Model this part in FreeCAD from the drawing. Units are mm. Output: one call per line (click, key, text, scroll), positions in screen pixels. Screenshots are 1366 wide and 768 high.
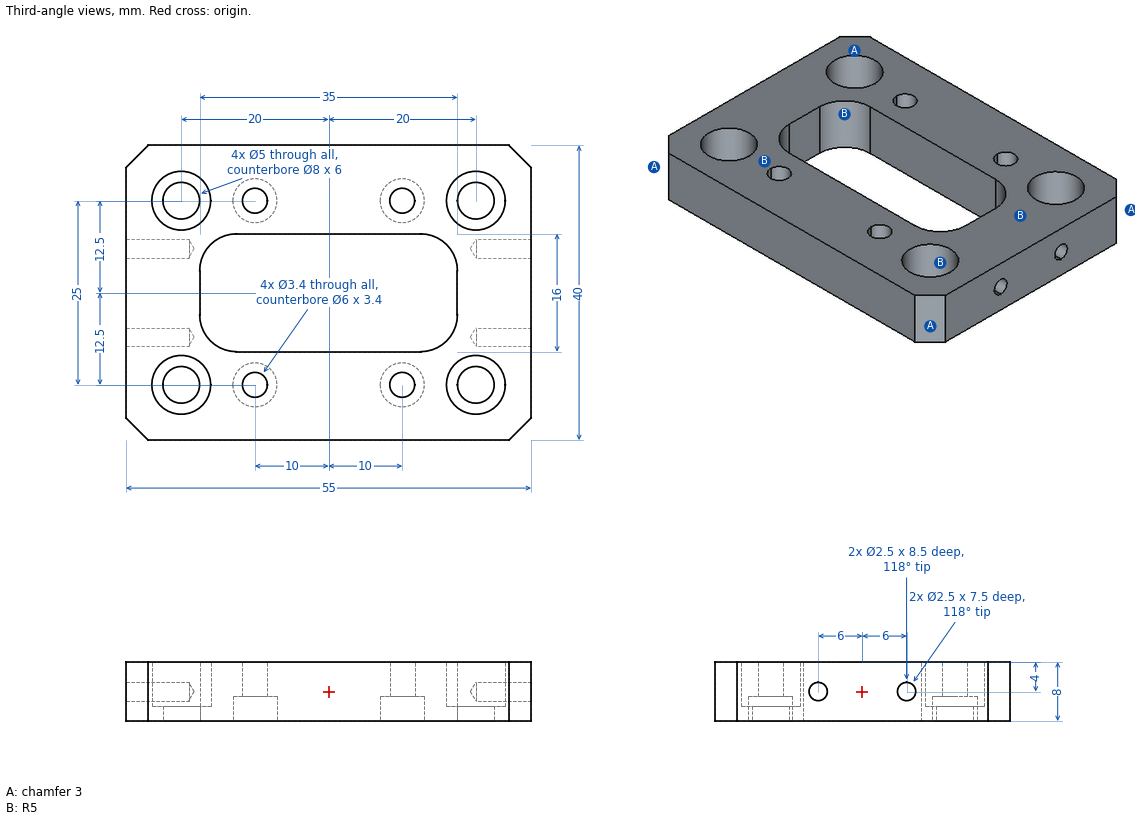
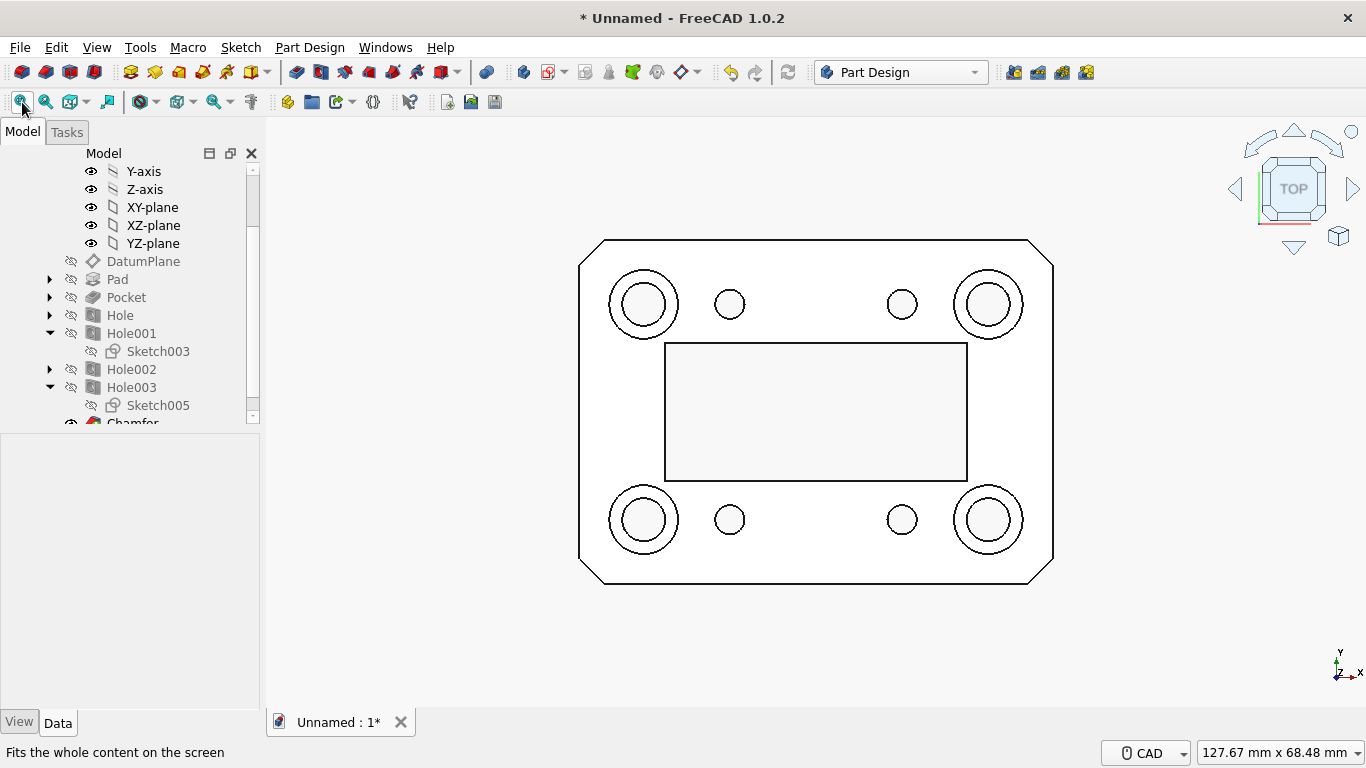
key(1)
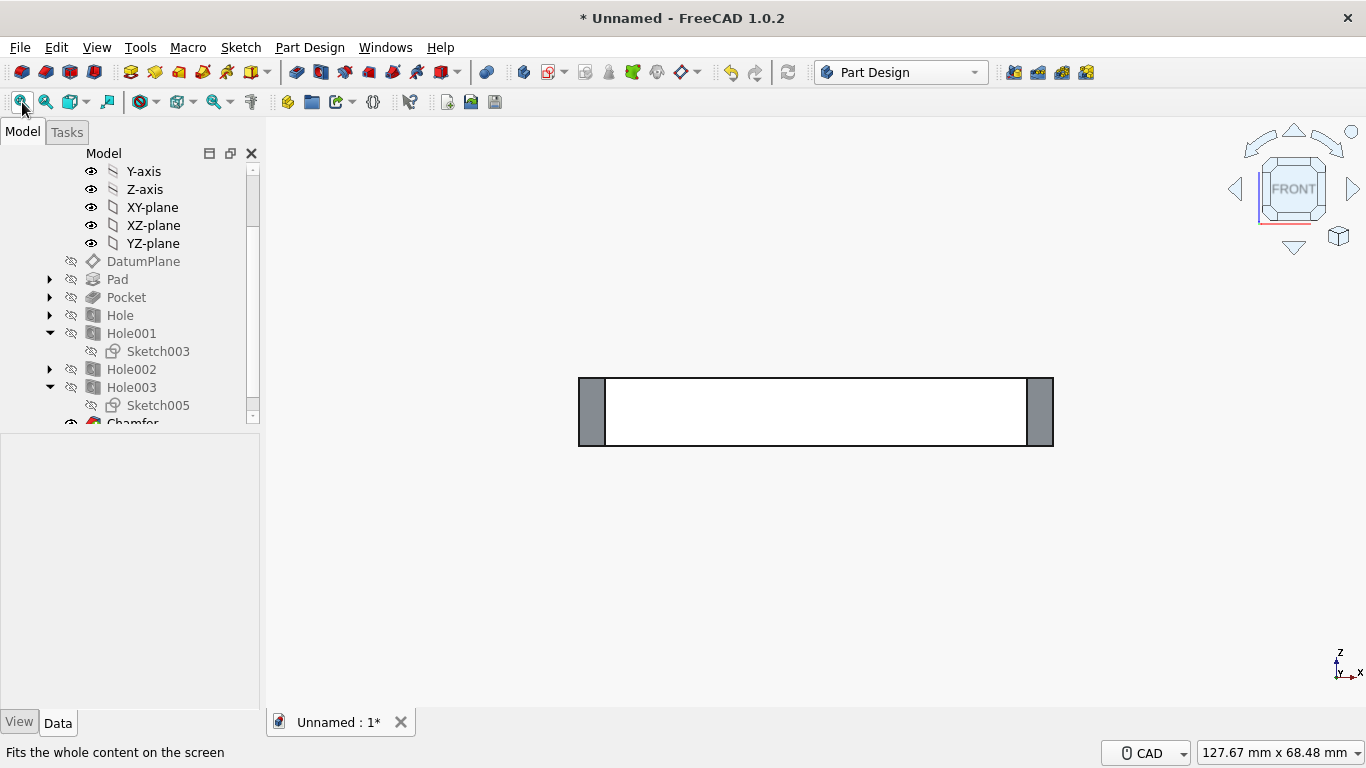
click(22, 102)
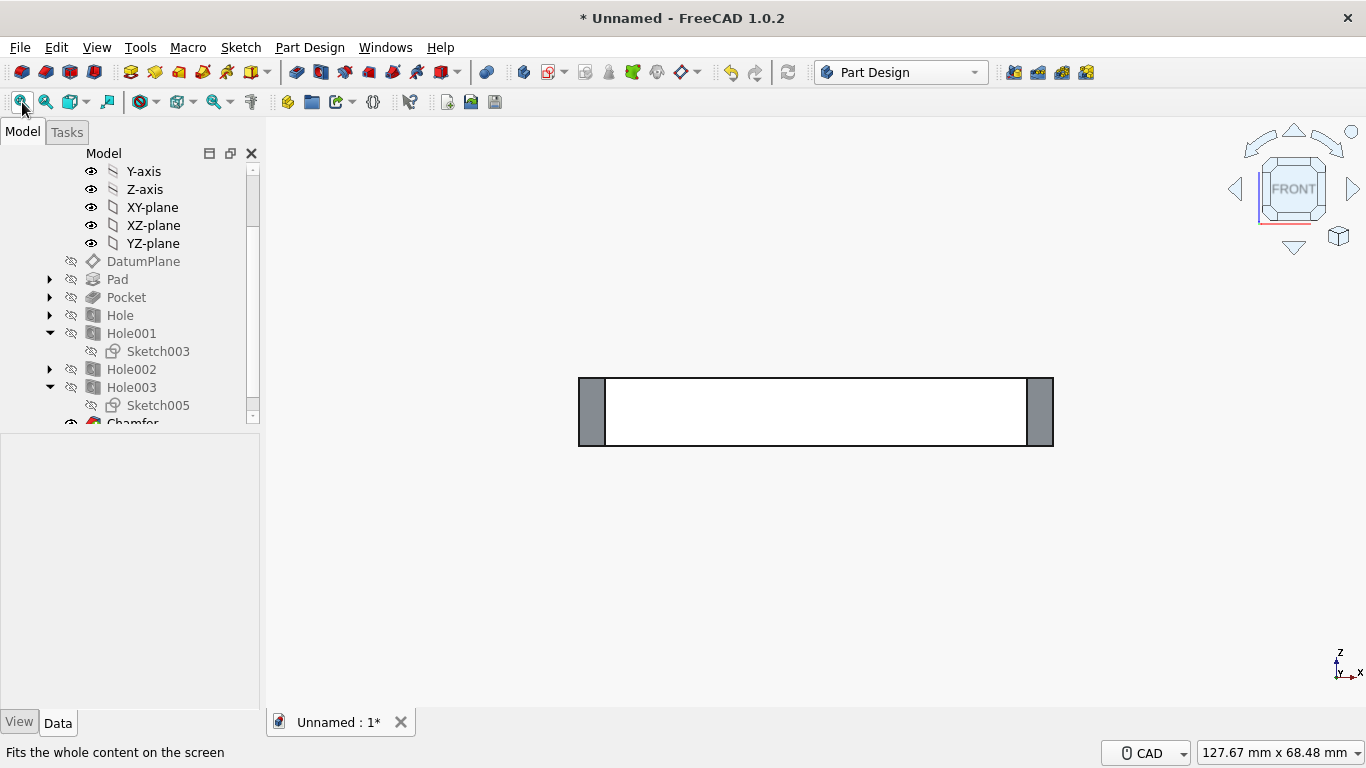
key(3)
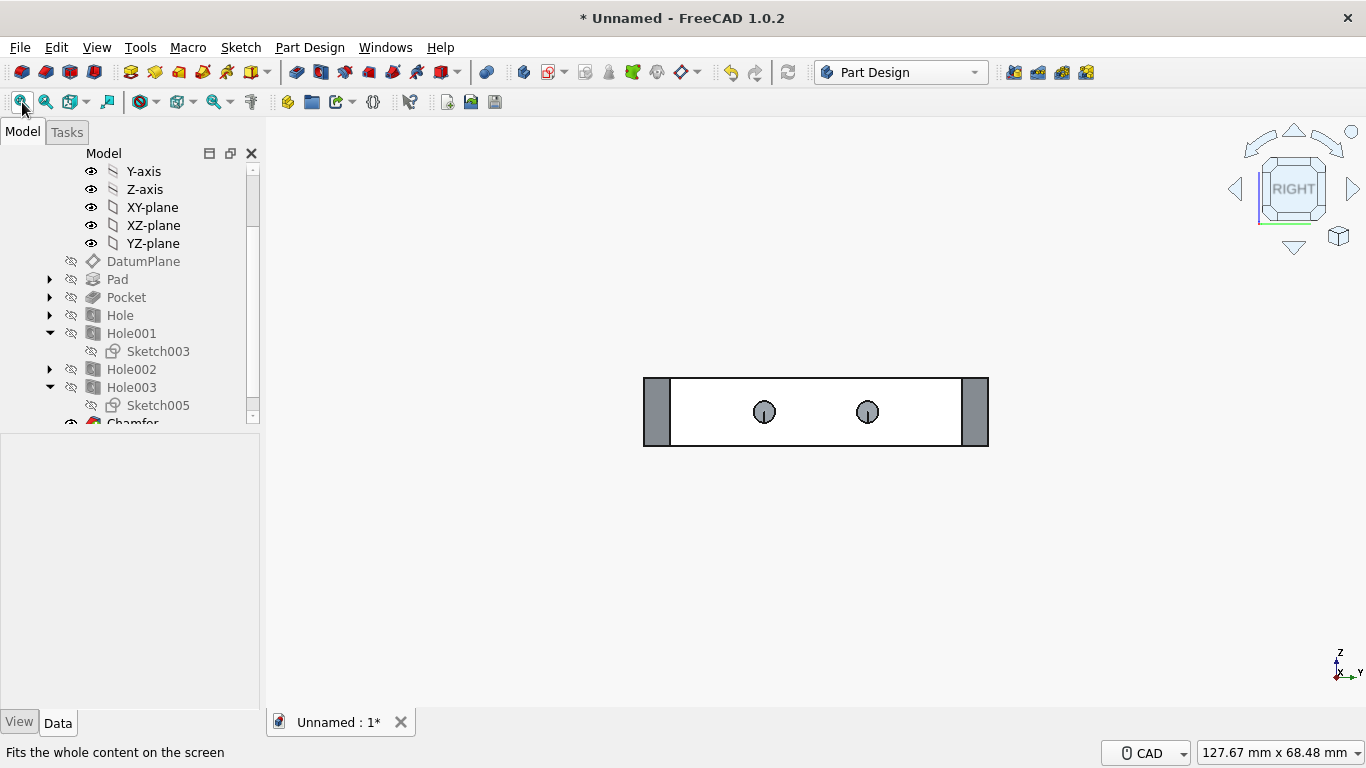
click(22, 102)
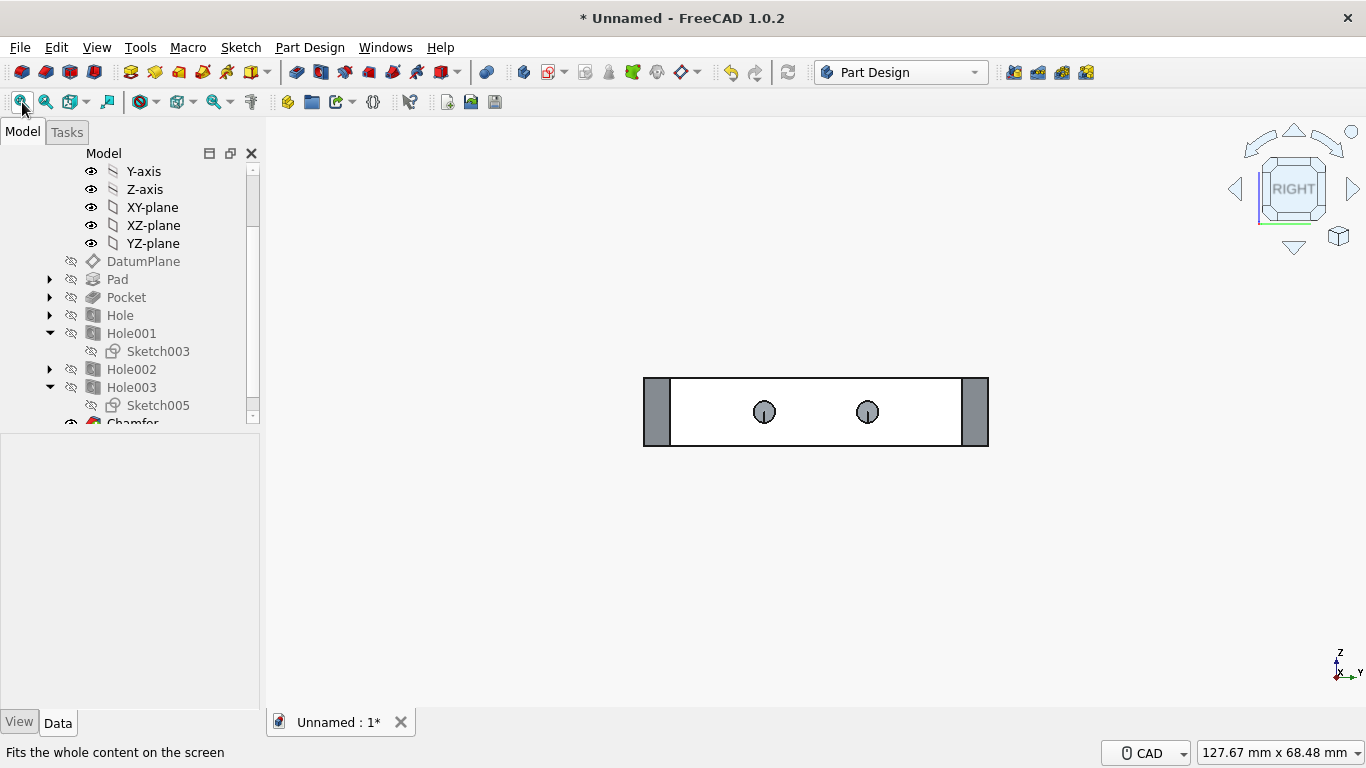
key(5)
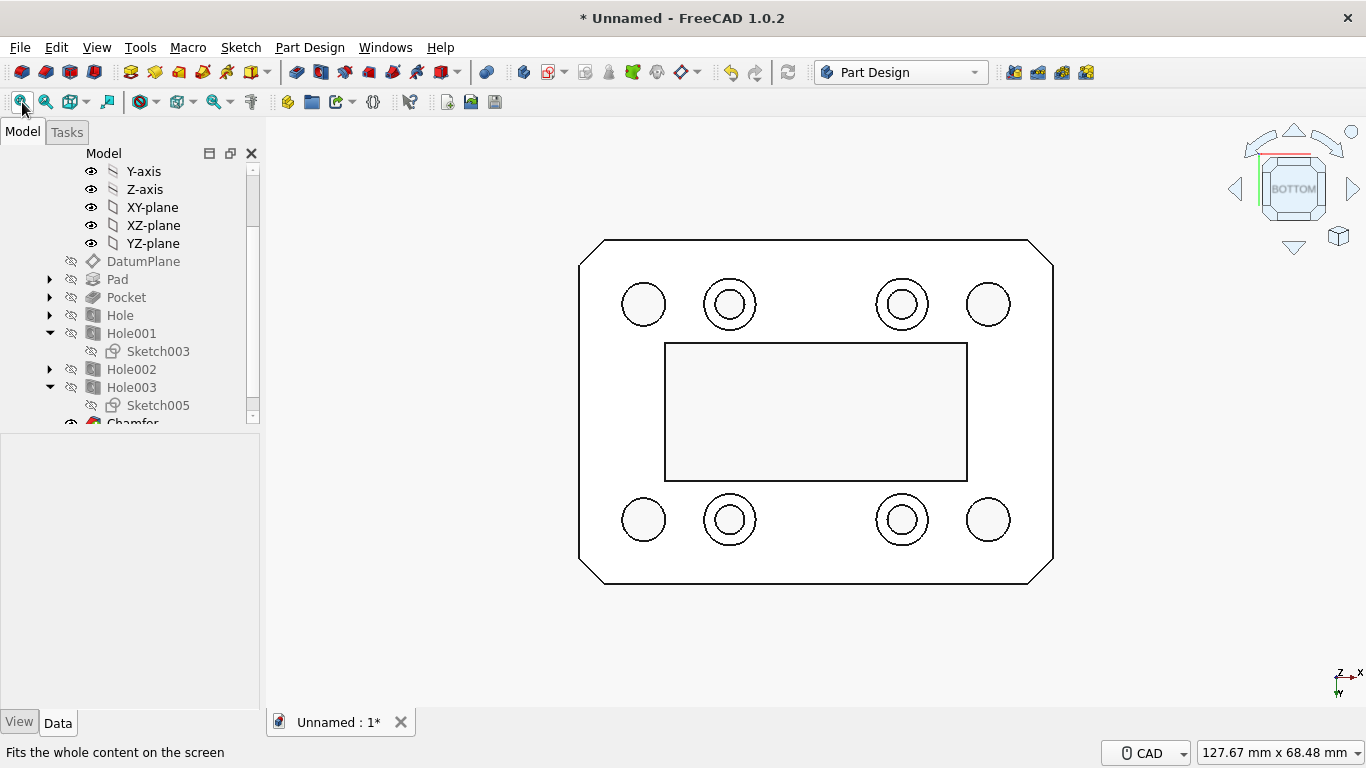
key(4)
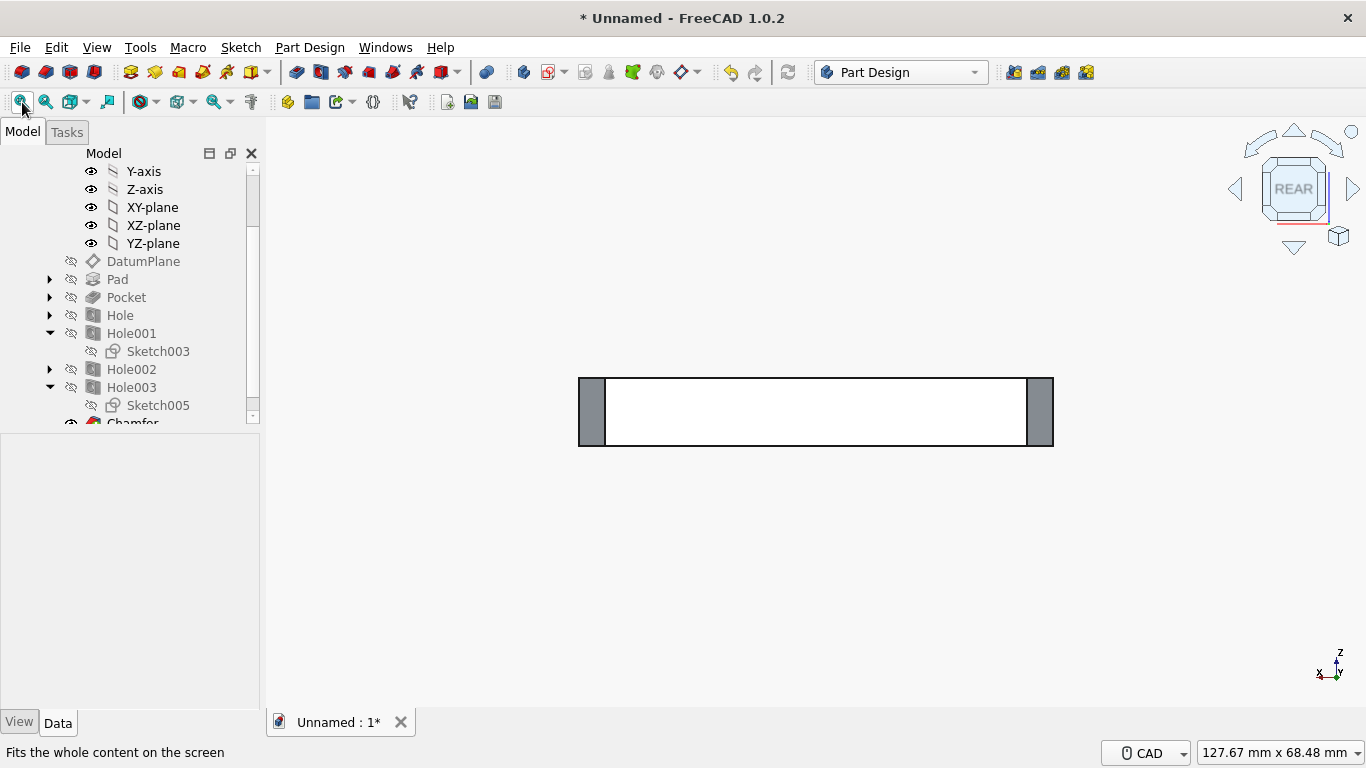
click(22, 102)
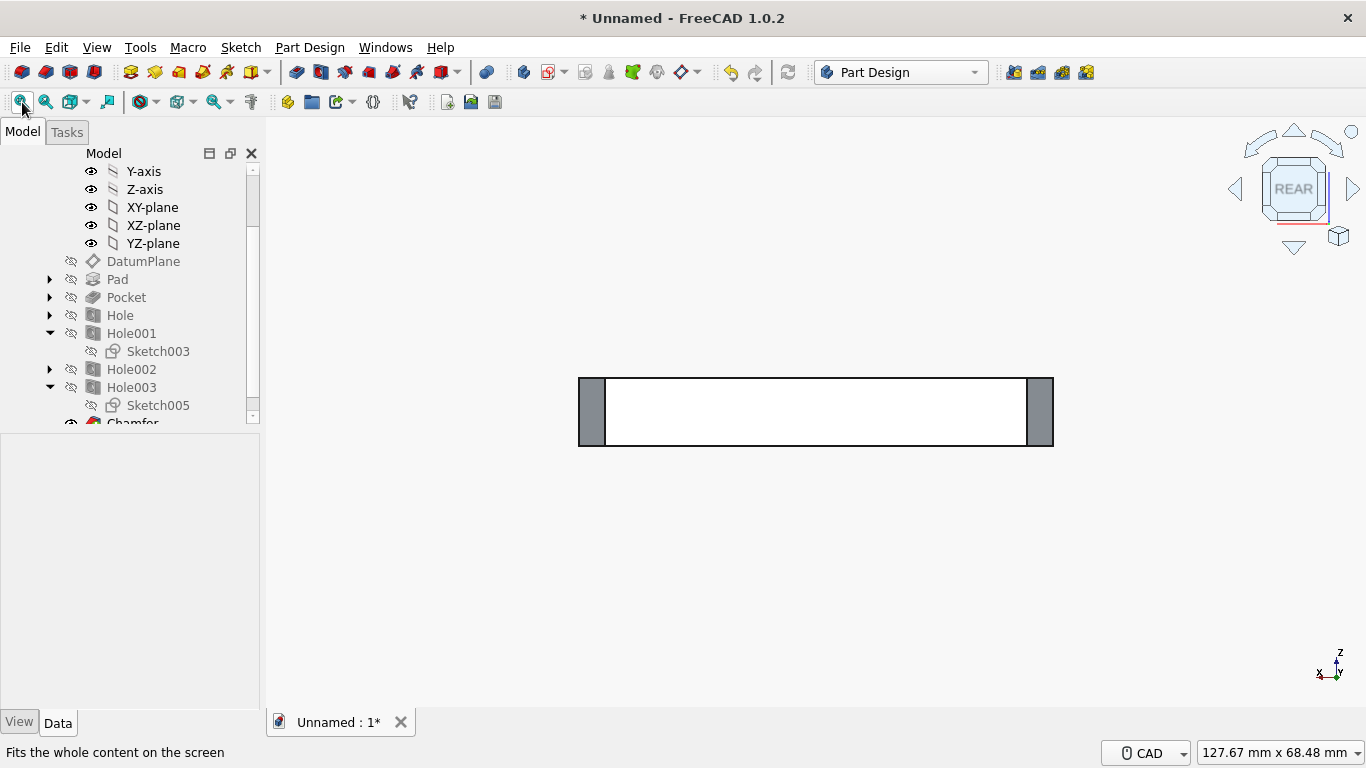
key(6)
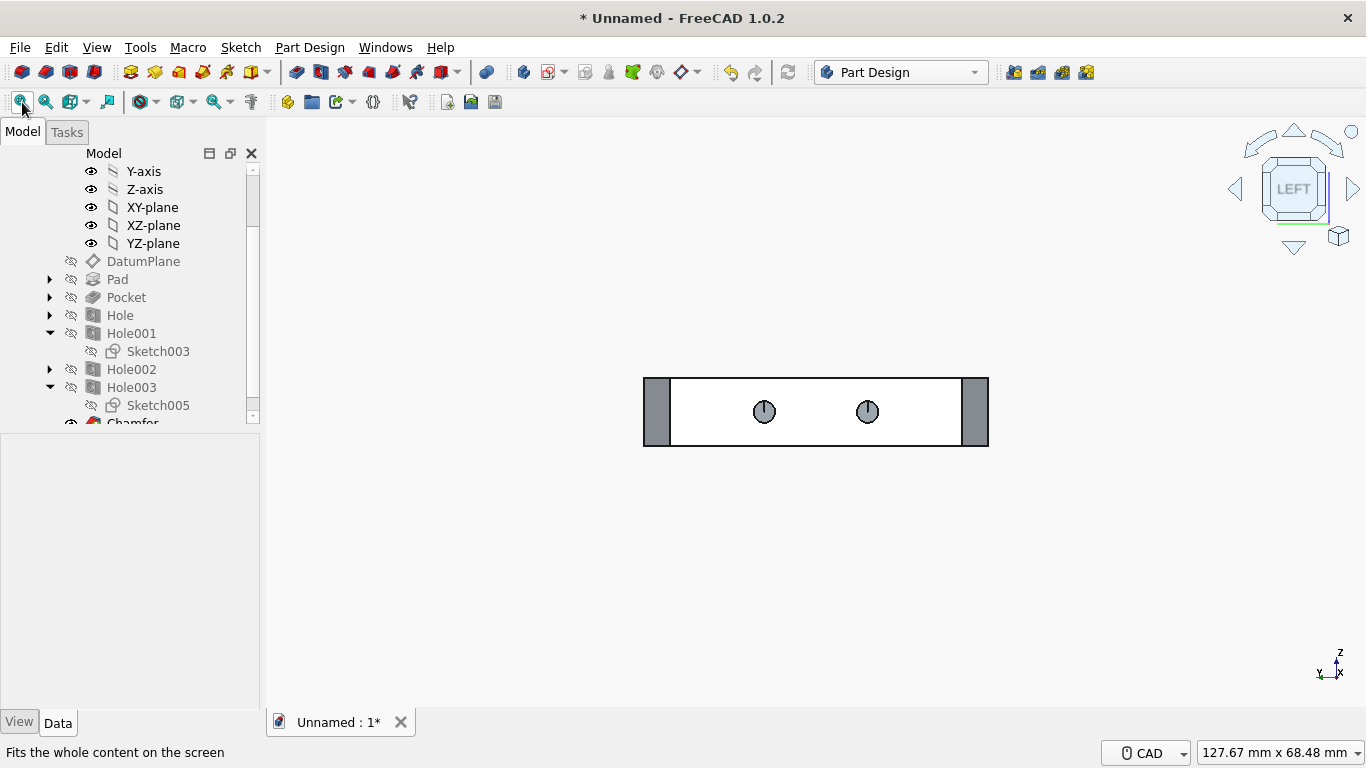
click(22, 102)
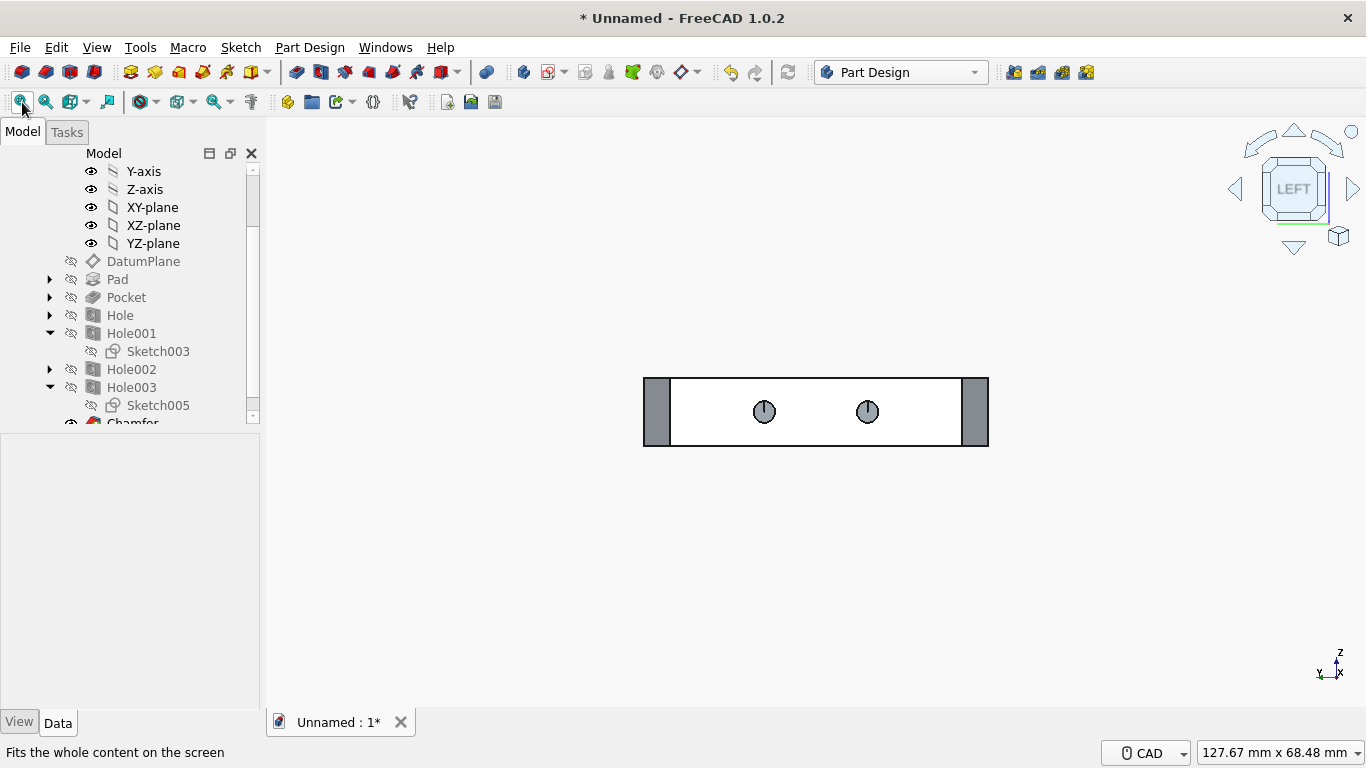
key(v)
key(3)